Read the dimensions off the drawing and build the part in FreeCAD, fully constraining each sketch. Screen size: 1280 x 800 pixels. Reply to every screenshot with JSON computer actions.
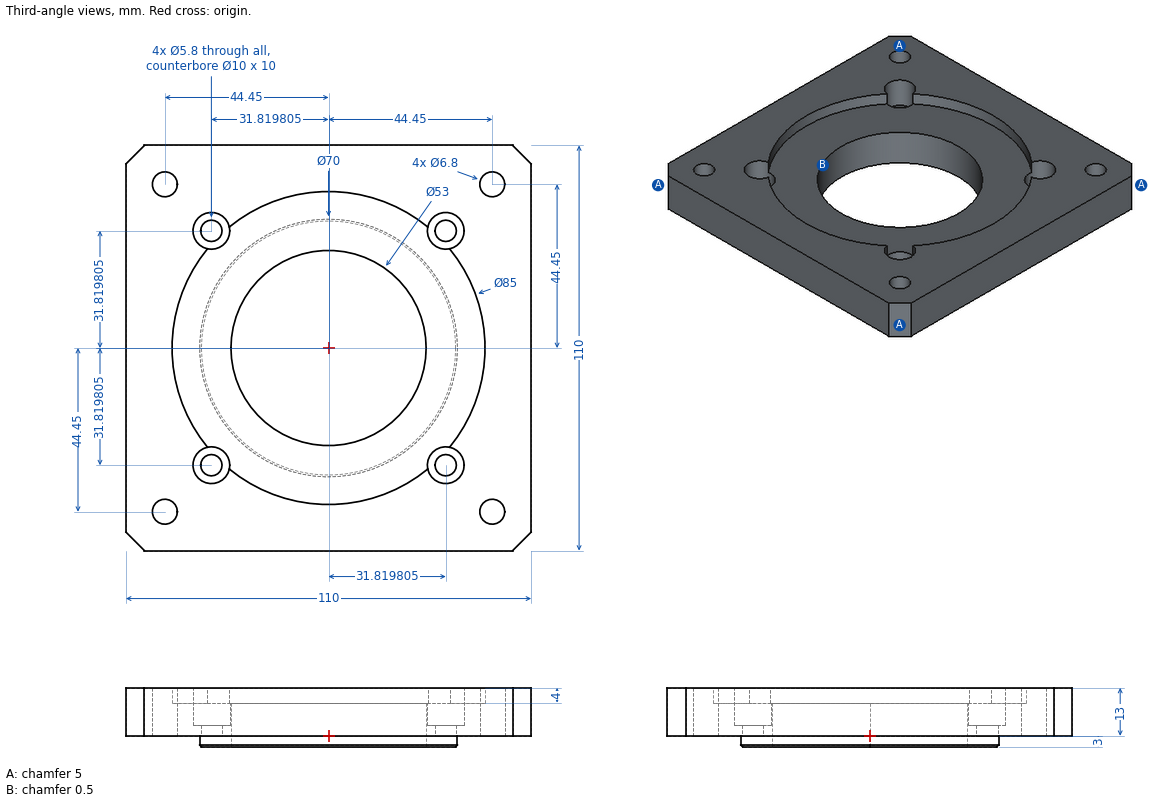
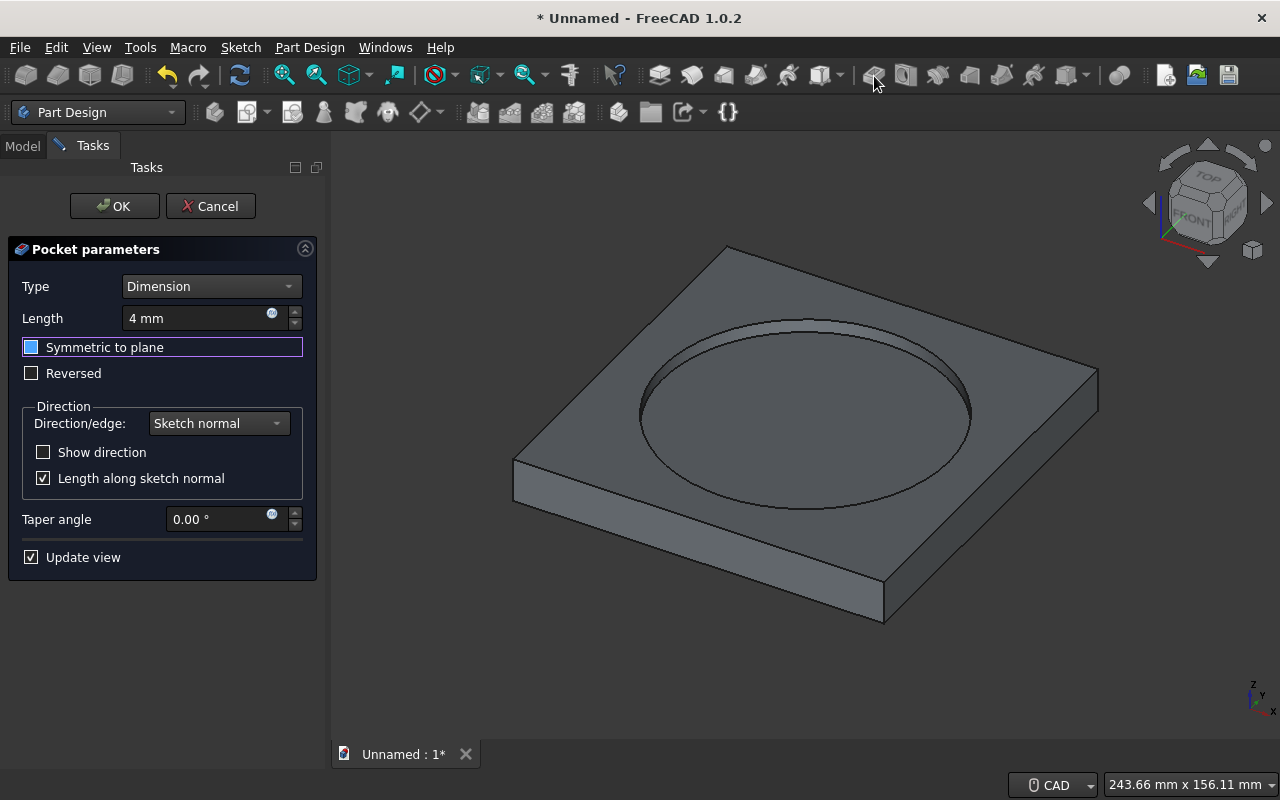
{"action": "left_click", "coordinate": [115, 206]}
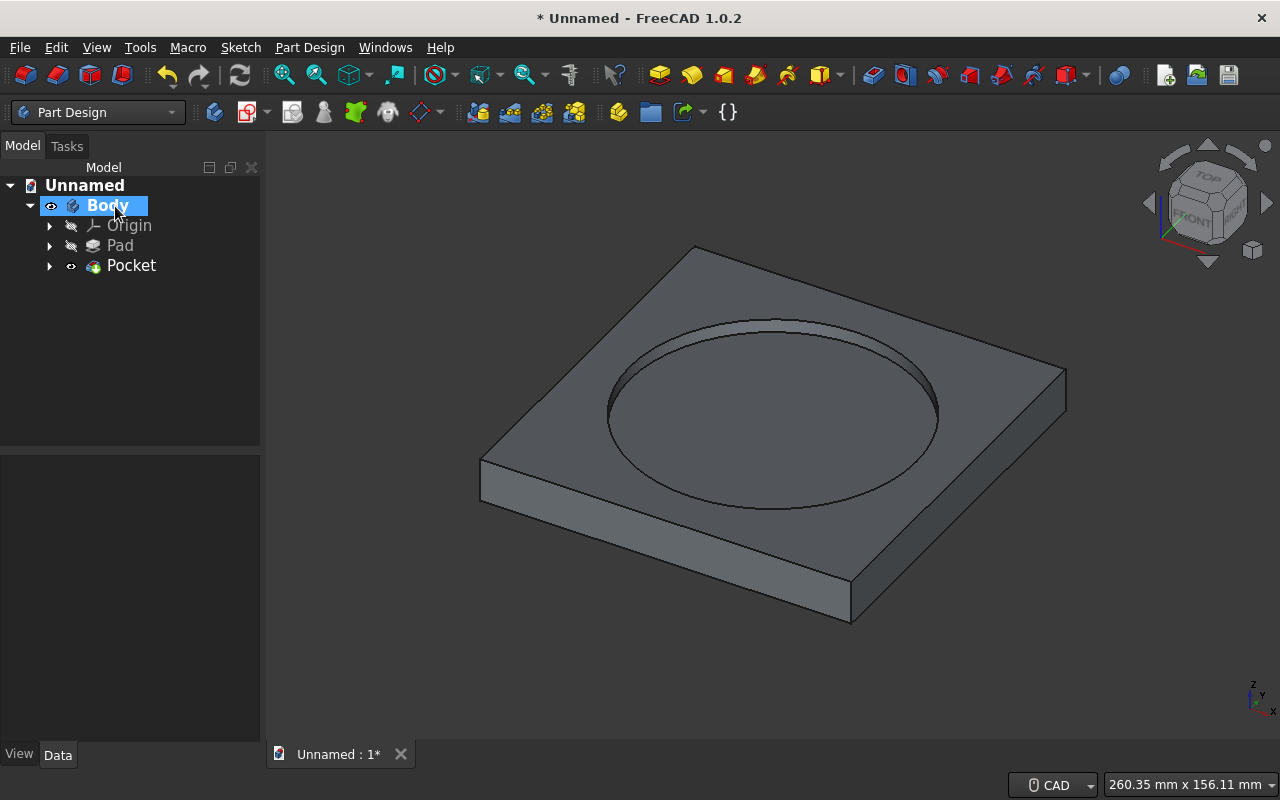
{"action": "left_click", "coordinate": [248, 112]}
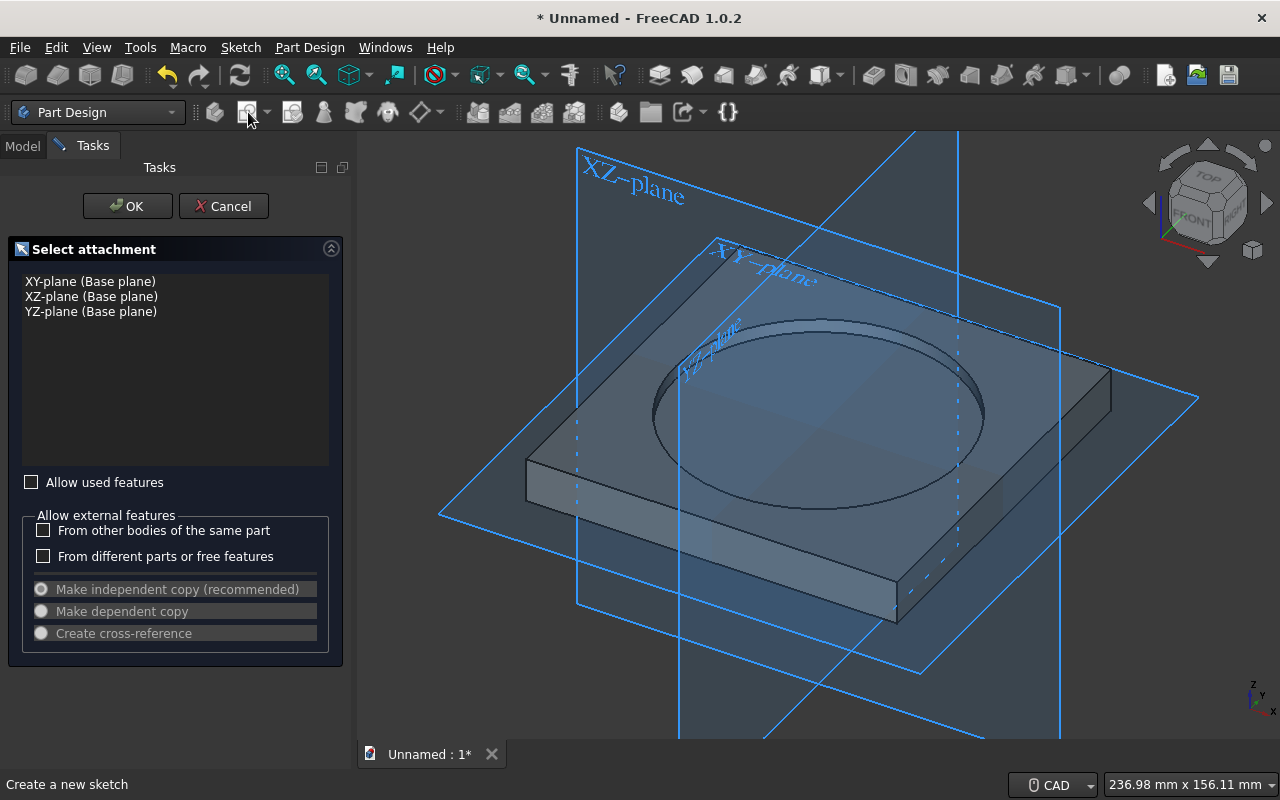
{"action": "left_click", "coordinate": [82, 282]}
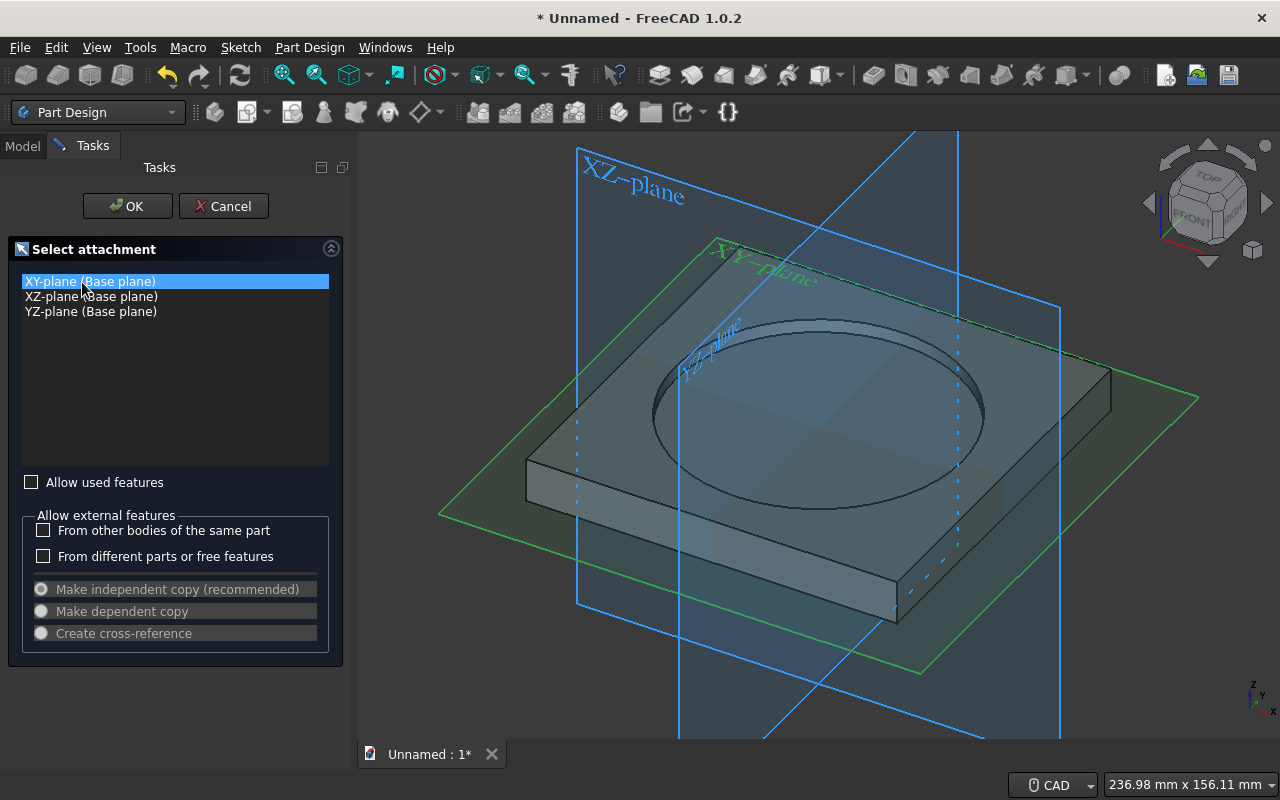
{"action": "left_click", "coordinate": [128, 206]}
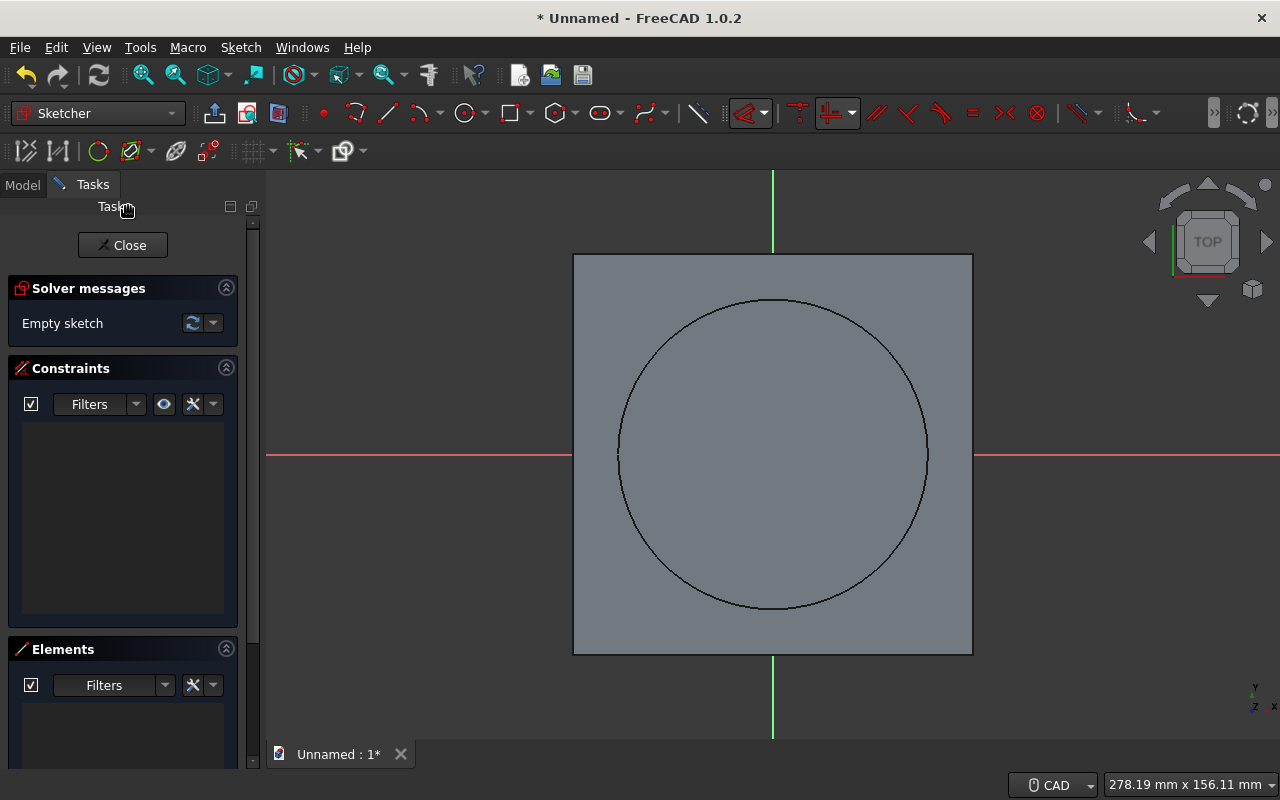
{"action": "left_click", "coordinate": [280, 114]}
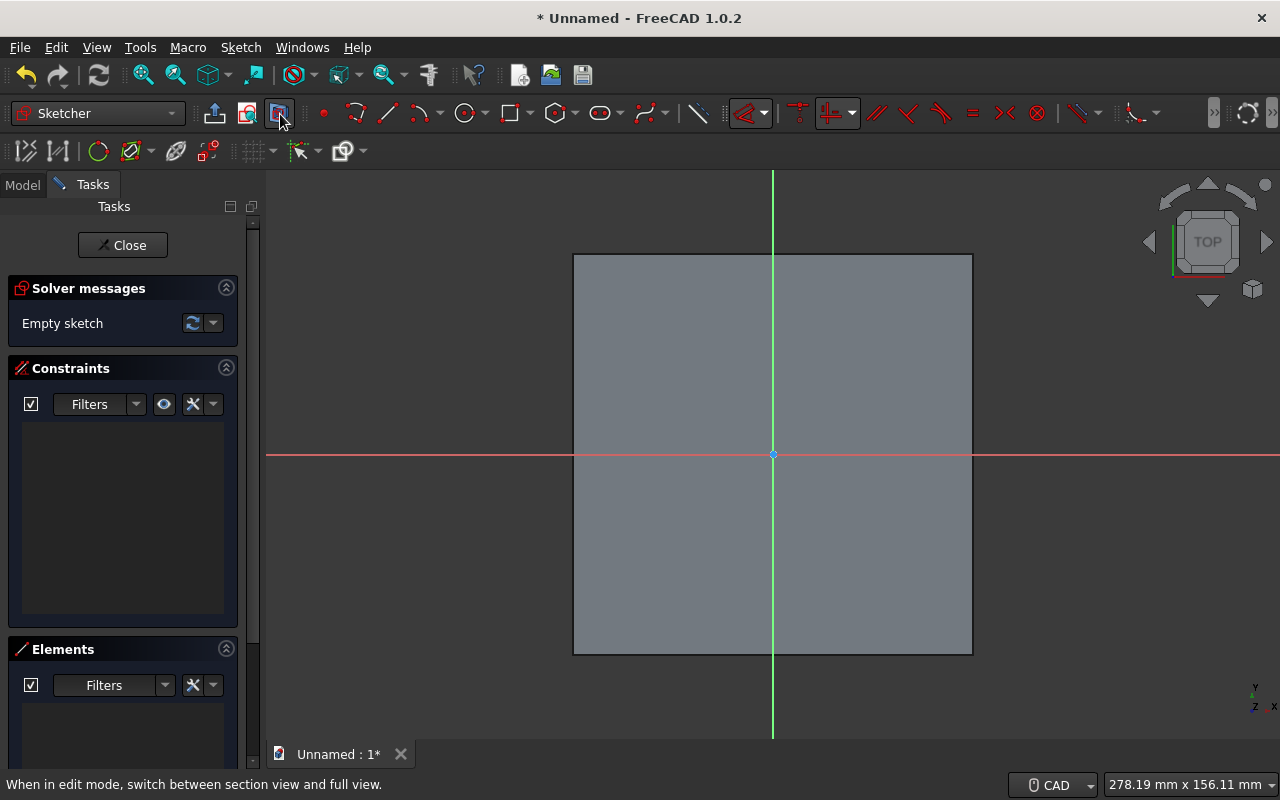
{"action": "scroll", "coordinate": [856, 455], "scroll_direction": "up", "scroll_amount": 3}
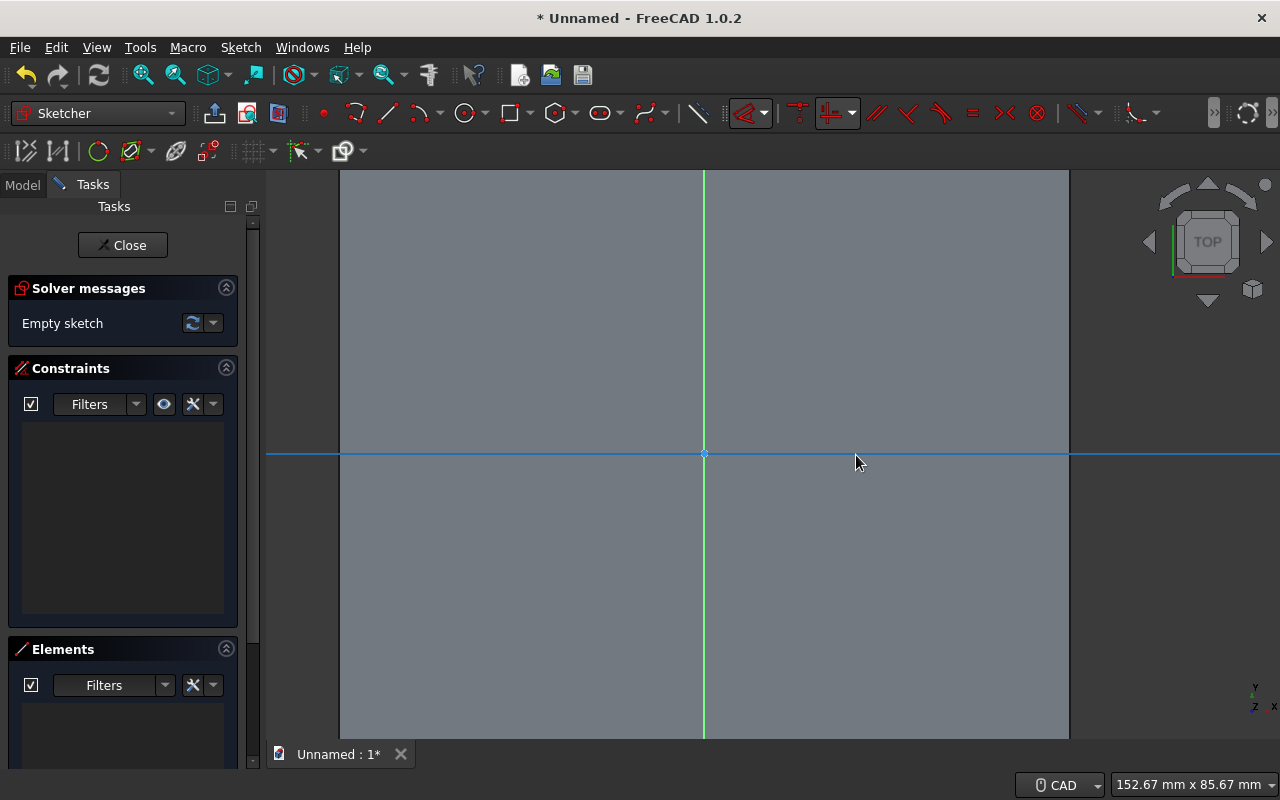
{"action": "left_click", "coordinate": [466, 114]}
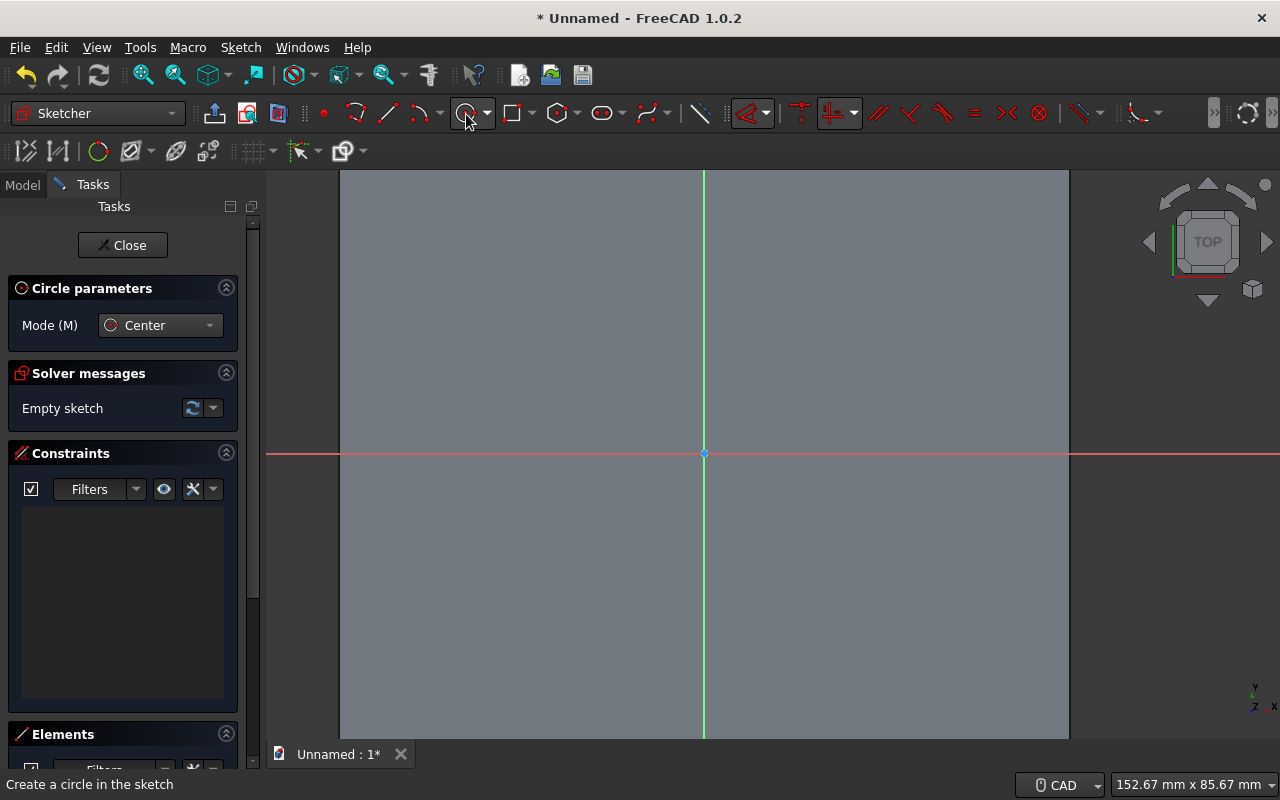
{"action": "left_click", "coordinate": [704, 454]}
{"action": "left_click", "coordinate": [829, 329]}
{"action": "key", "text": "Escape"}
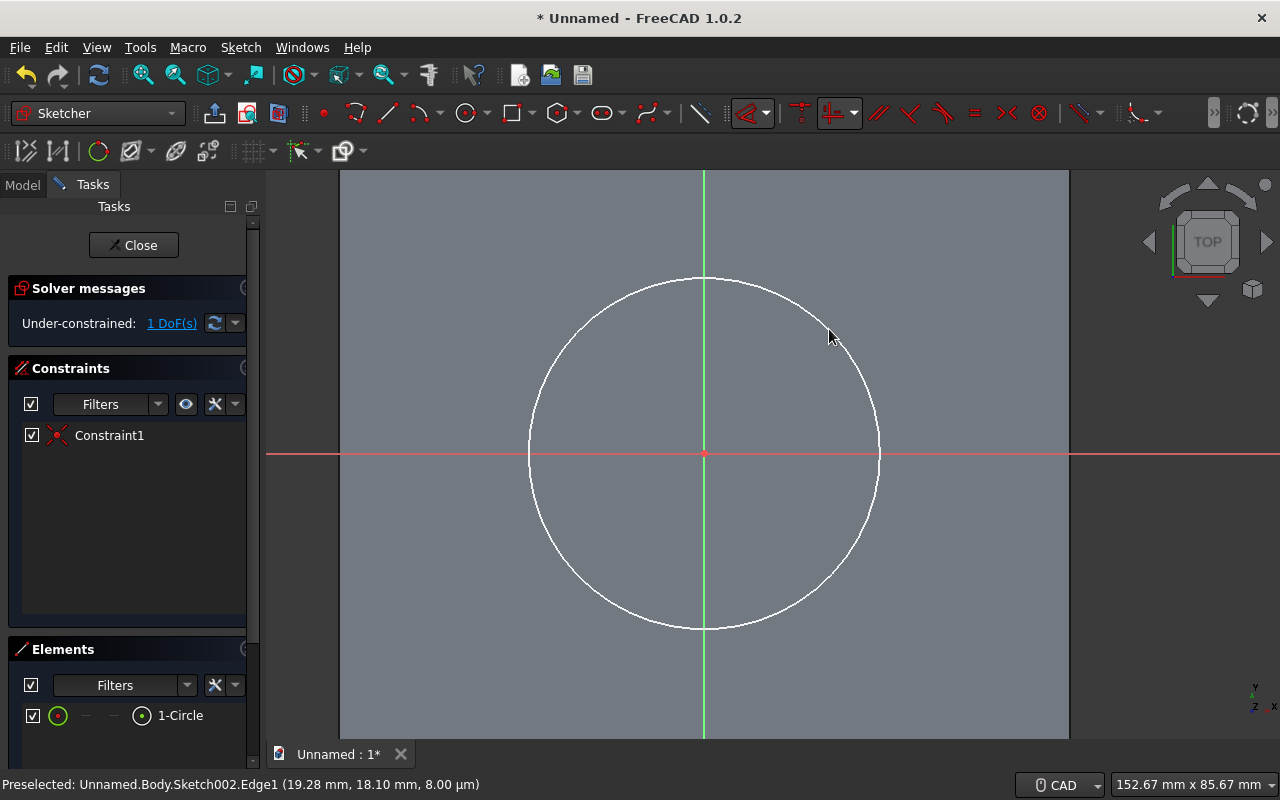
{"action": "left_click", "coordinate": [828, 329]}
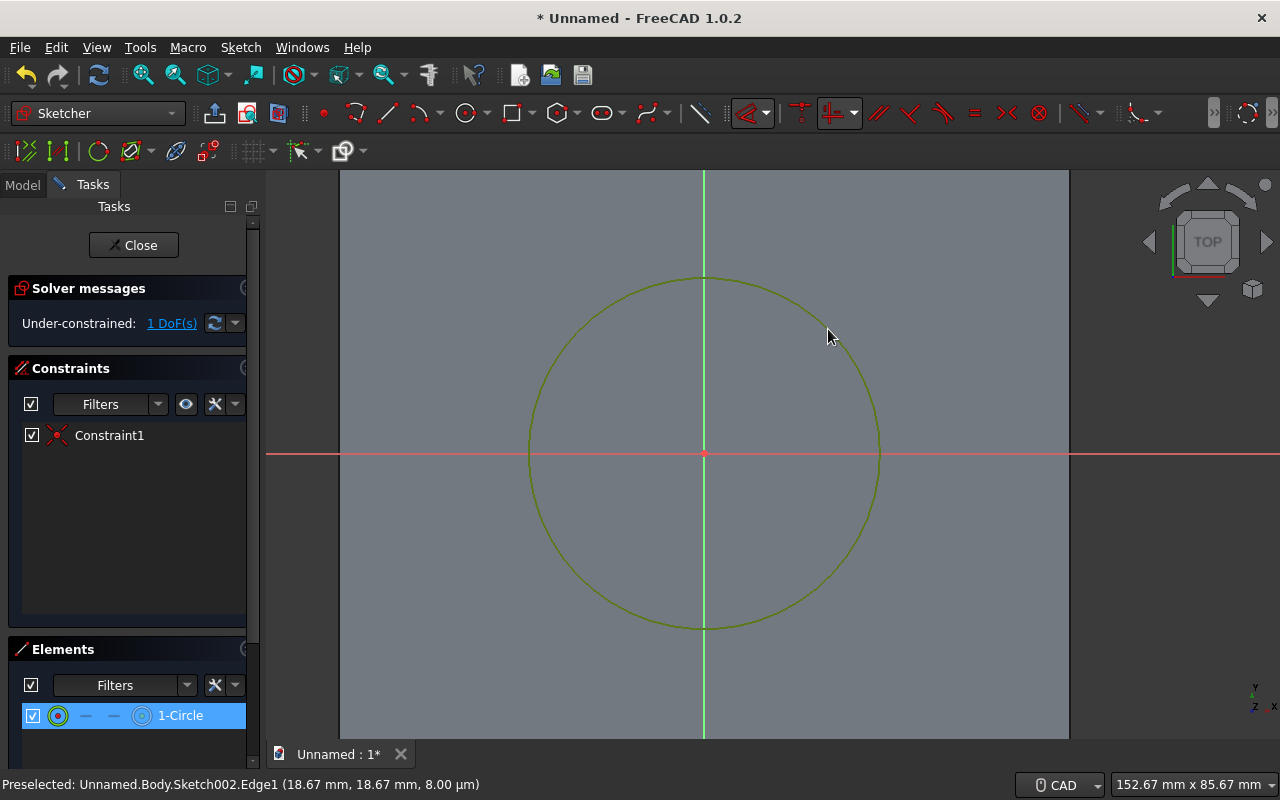
{"action": "key", "text": "k o"}